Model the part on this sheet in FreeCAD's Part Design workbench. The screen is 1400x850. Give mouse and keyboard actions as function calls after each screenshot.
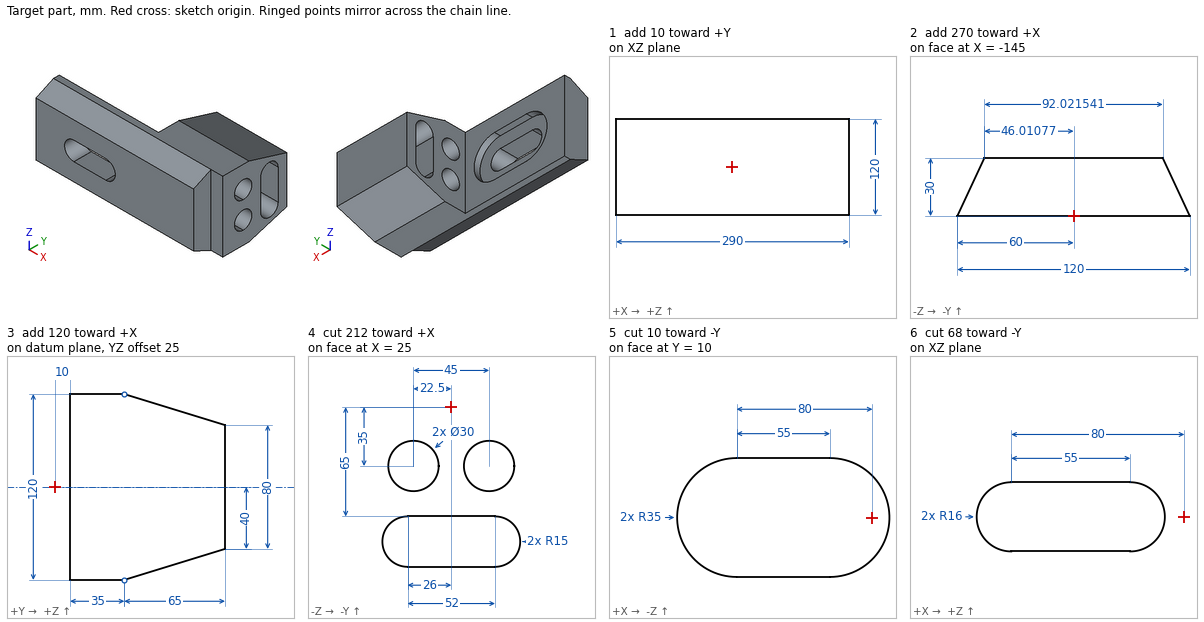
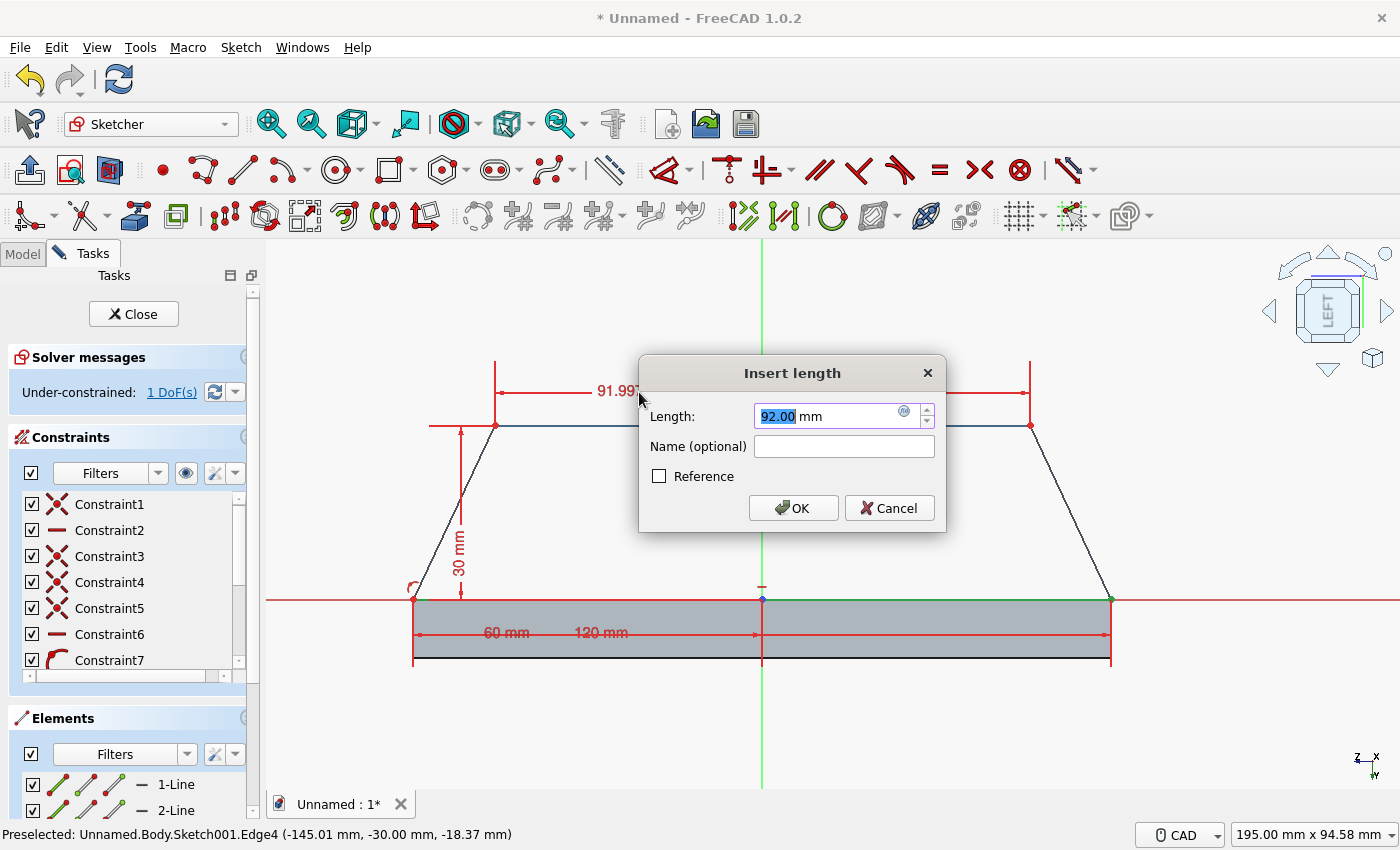
text(92.021541)
key(Return)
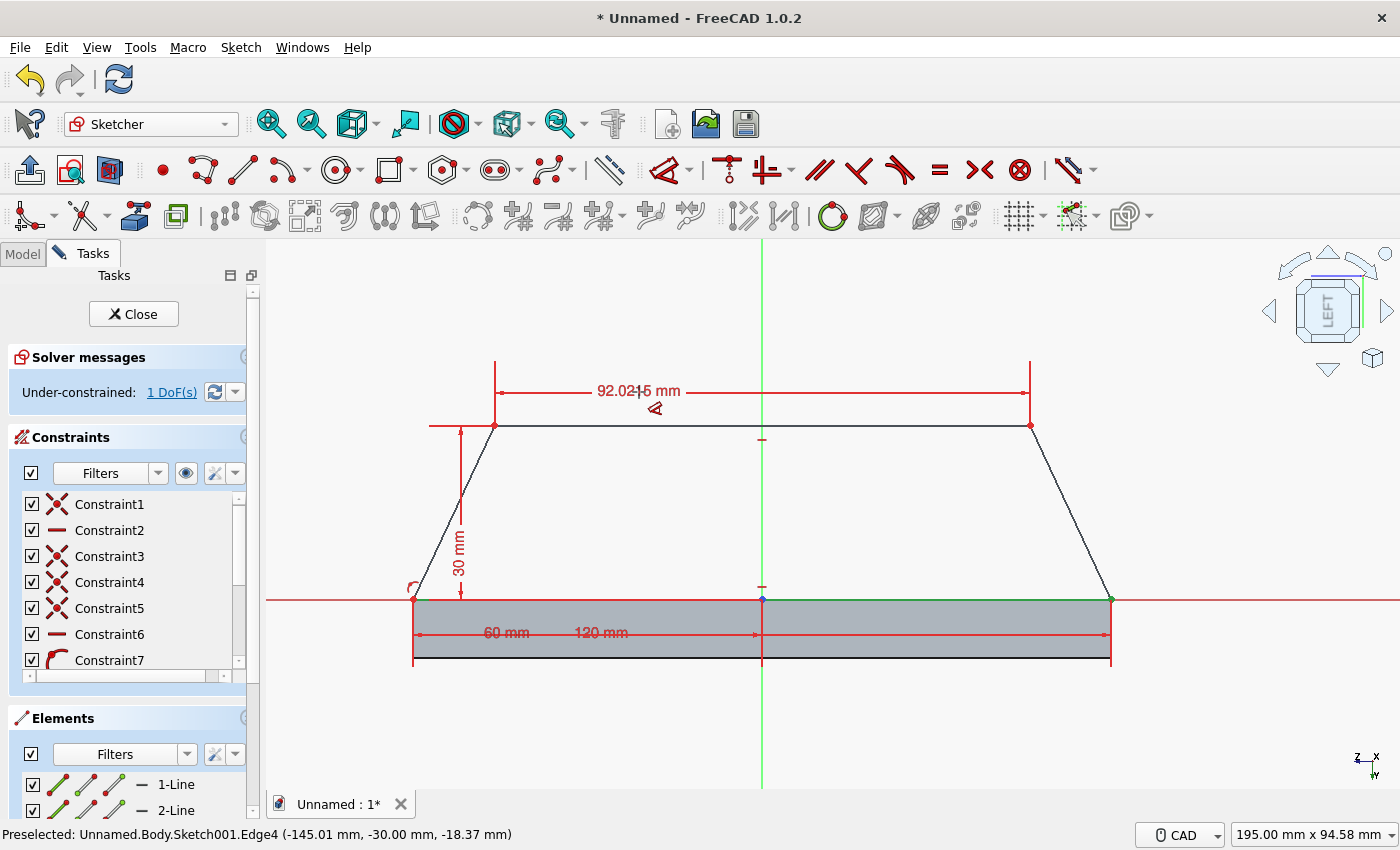
click(495, 426)
click(690, 634)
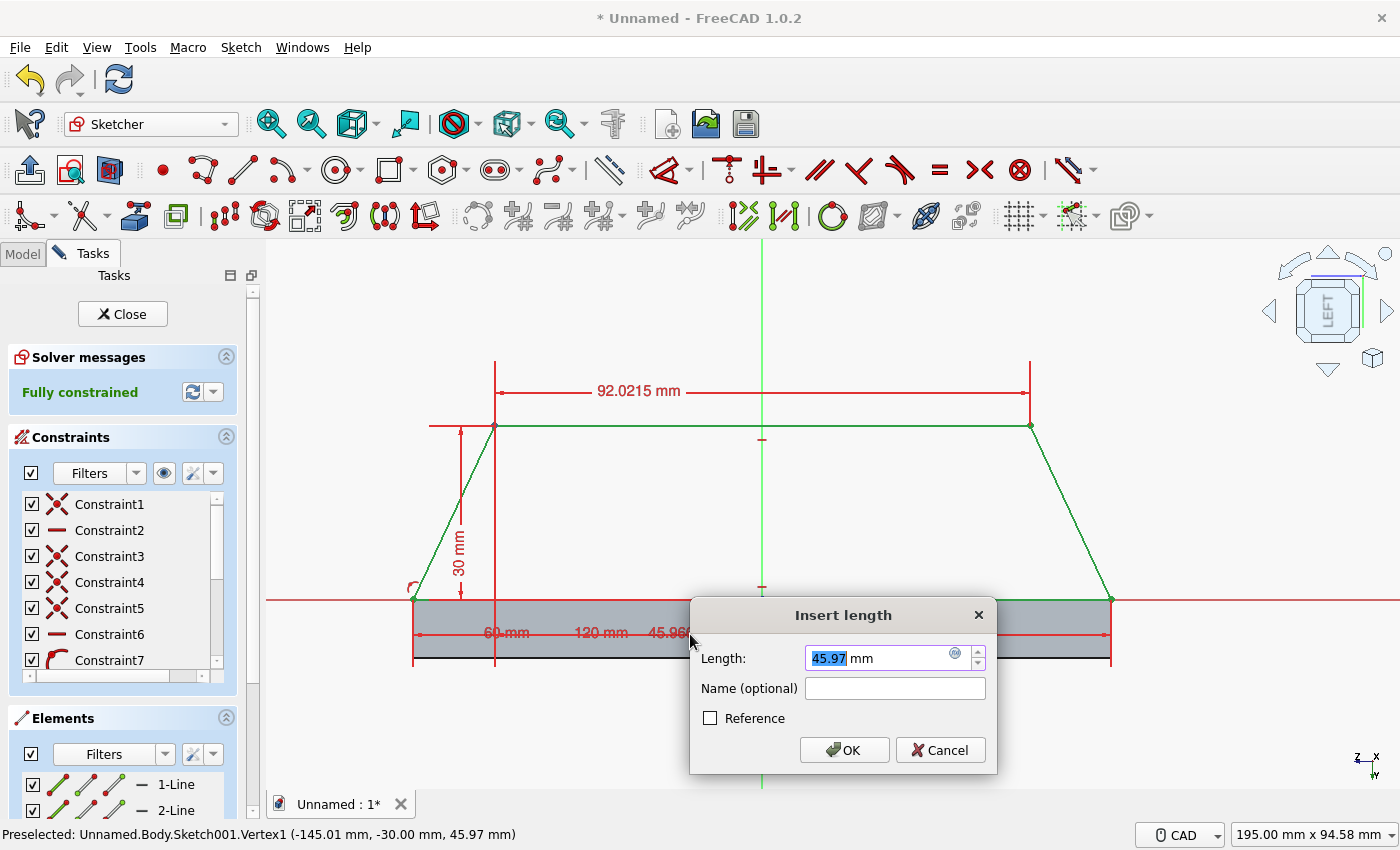
text(46.01077)
key(Return)
key(Escape)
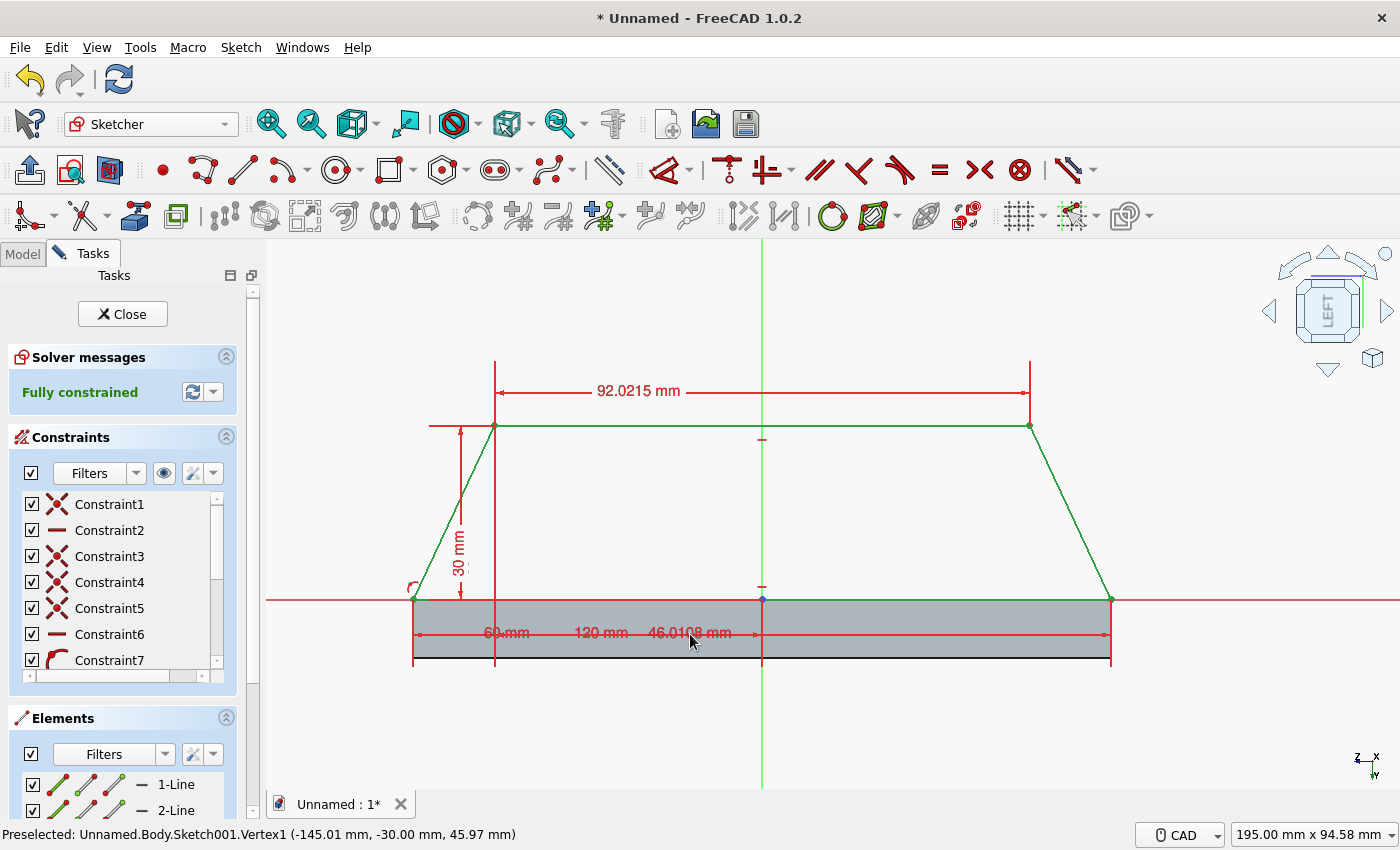
click(123, 314)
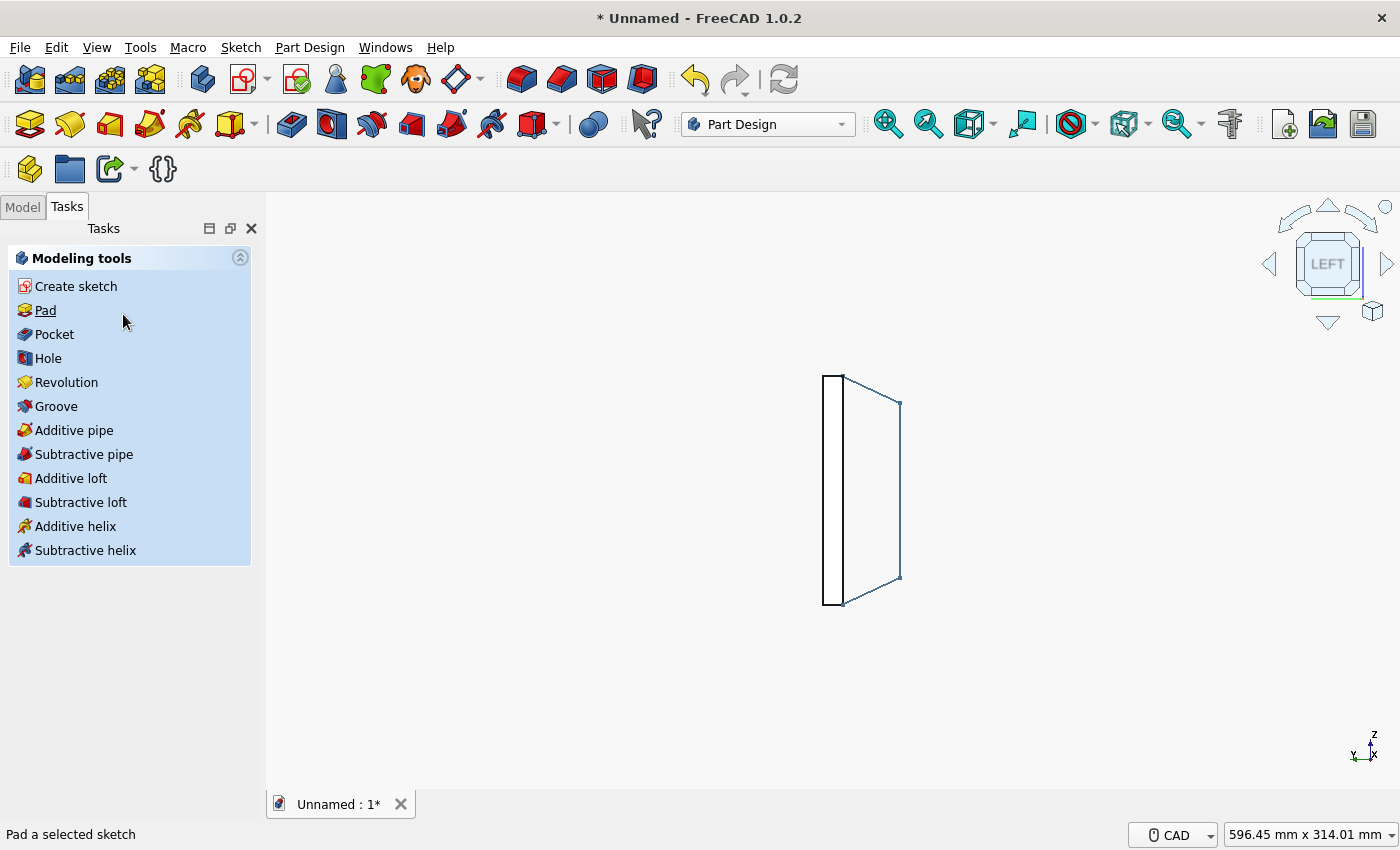
click(30, 124)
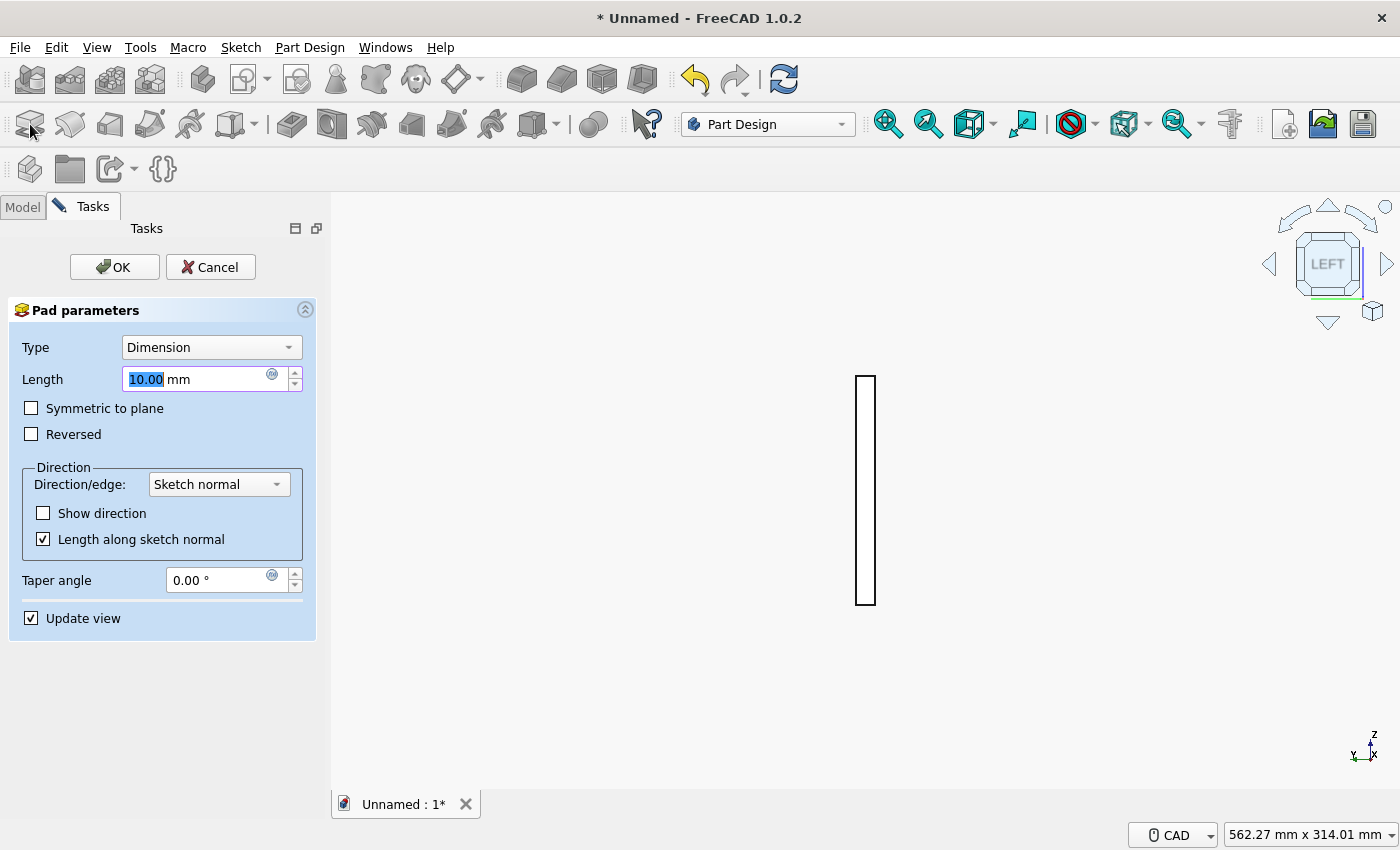
text(270)
key(Tab)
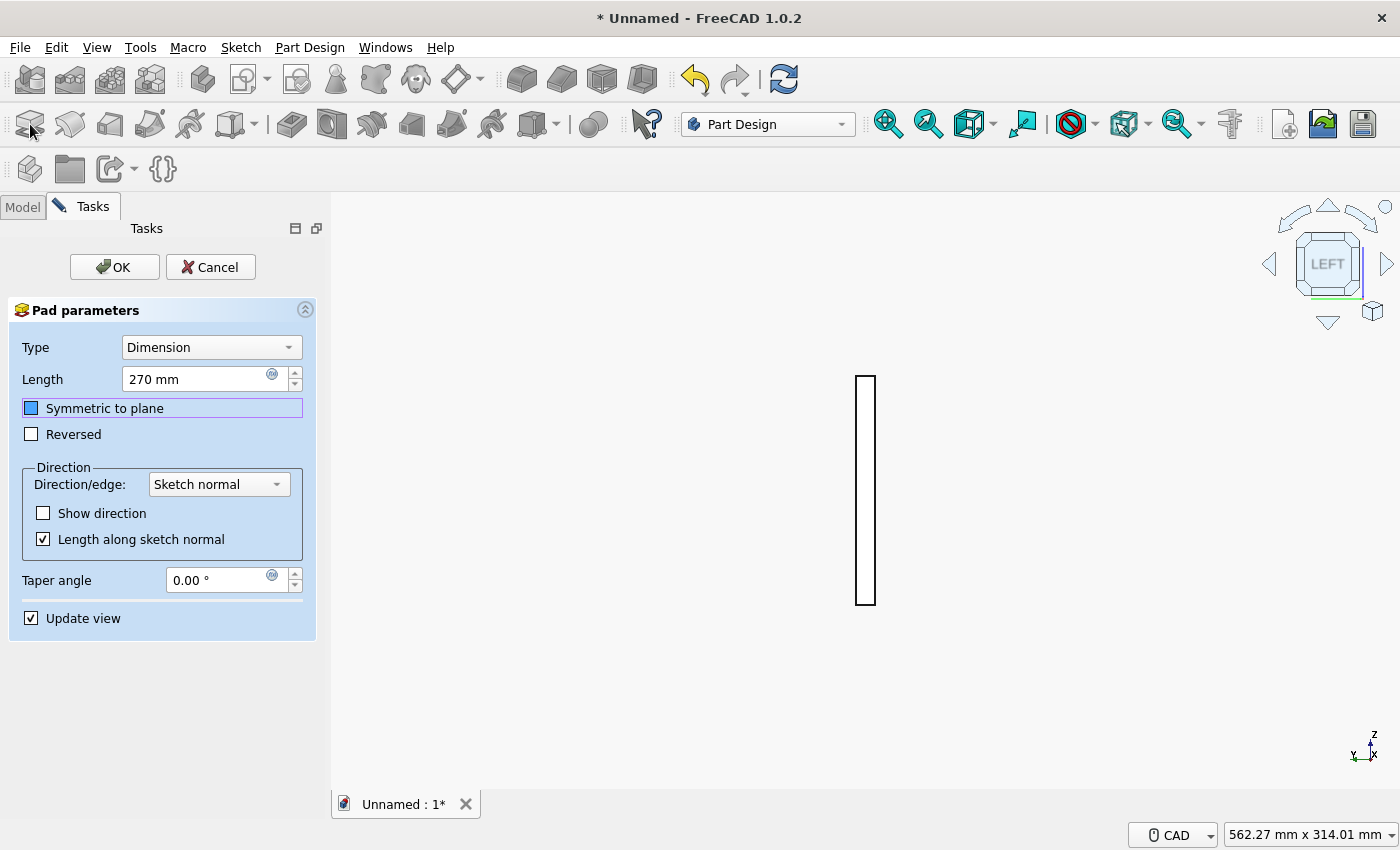
click(30, 434)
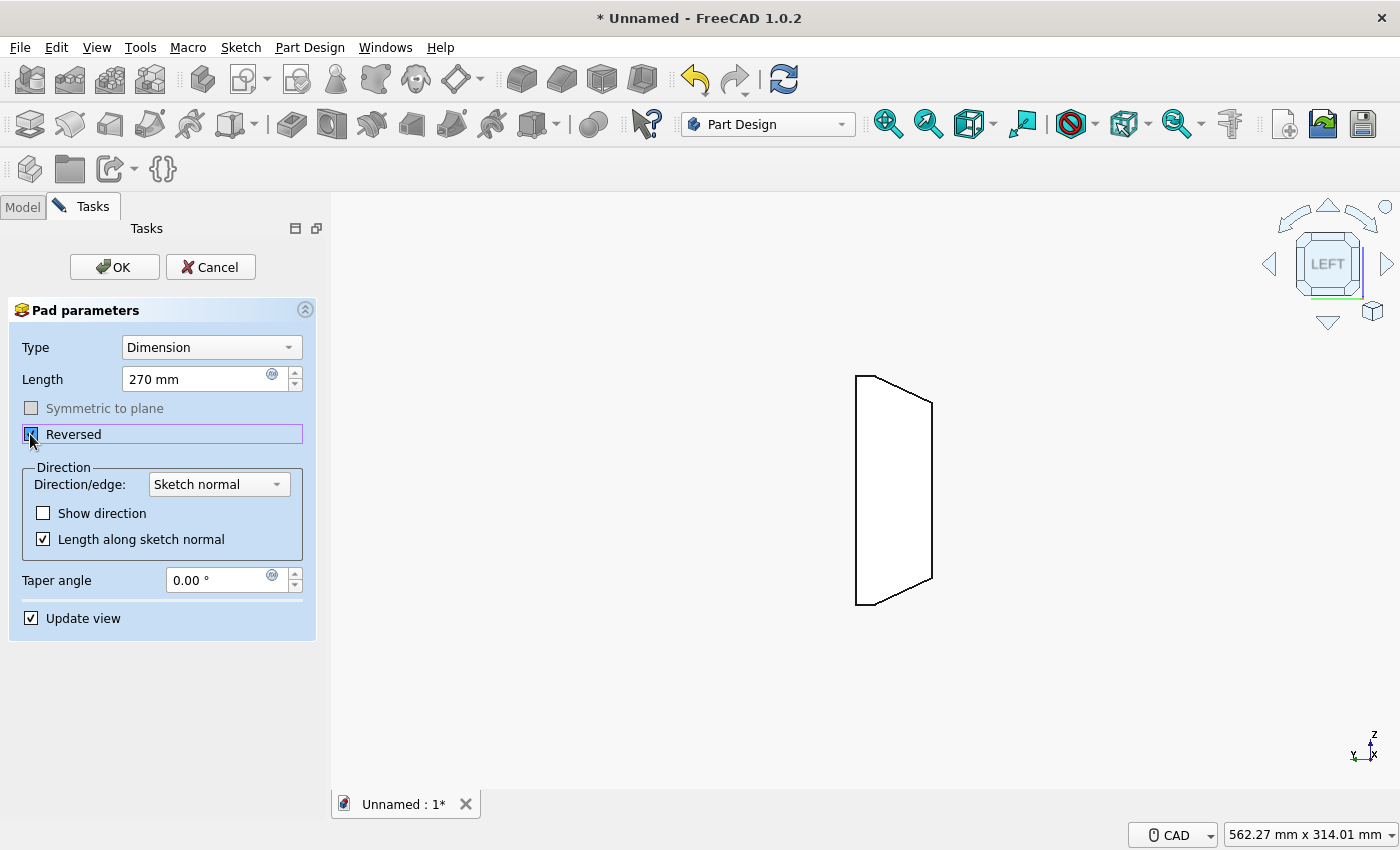
click(115, 267)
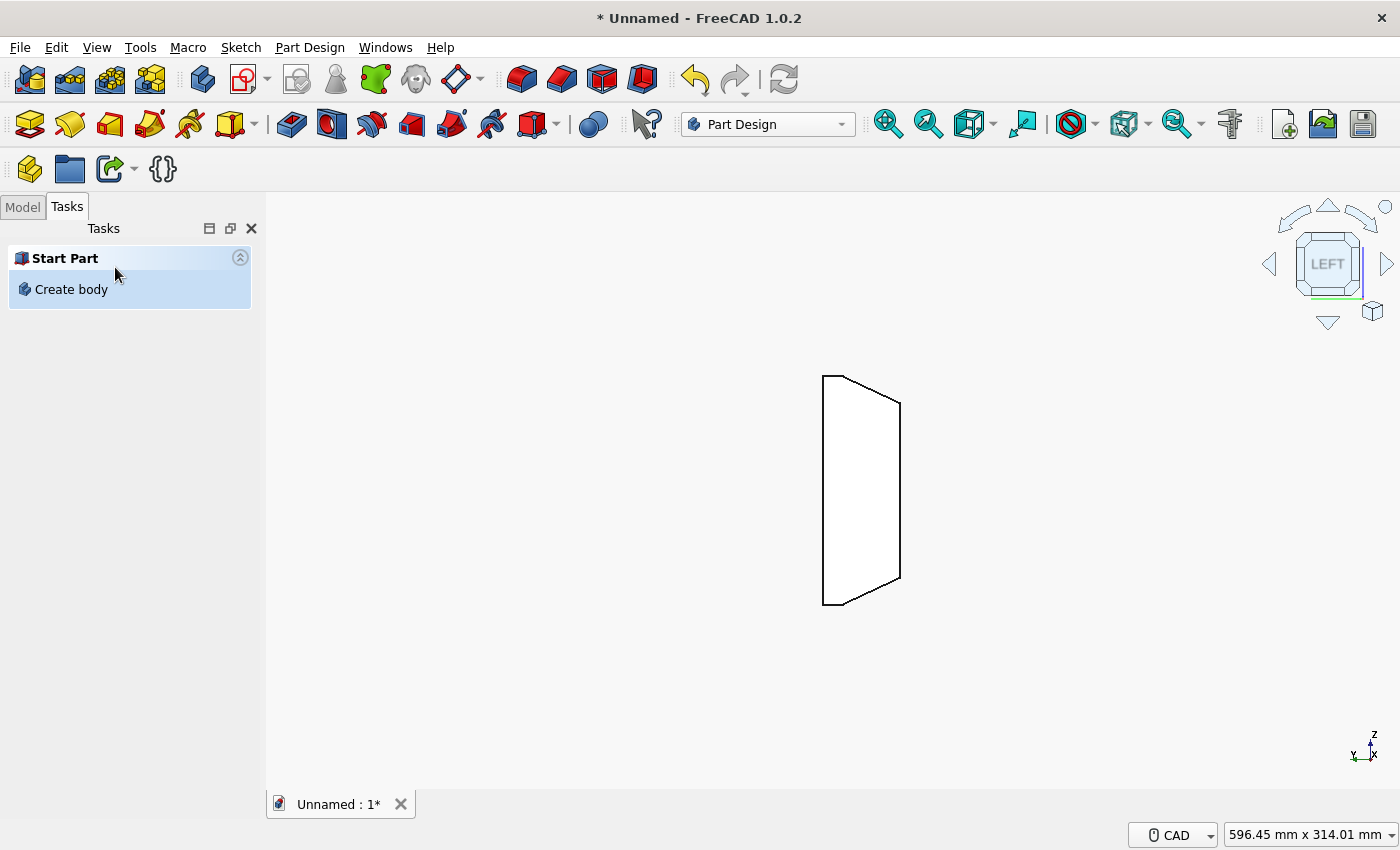
key(v)
key(f)